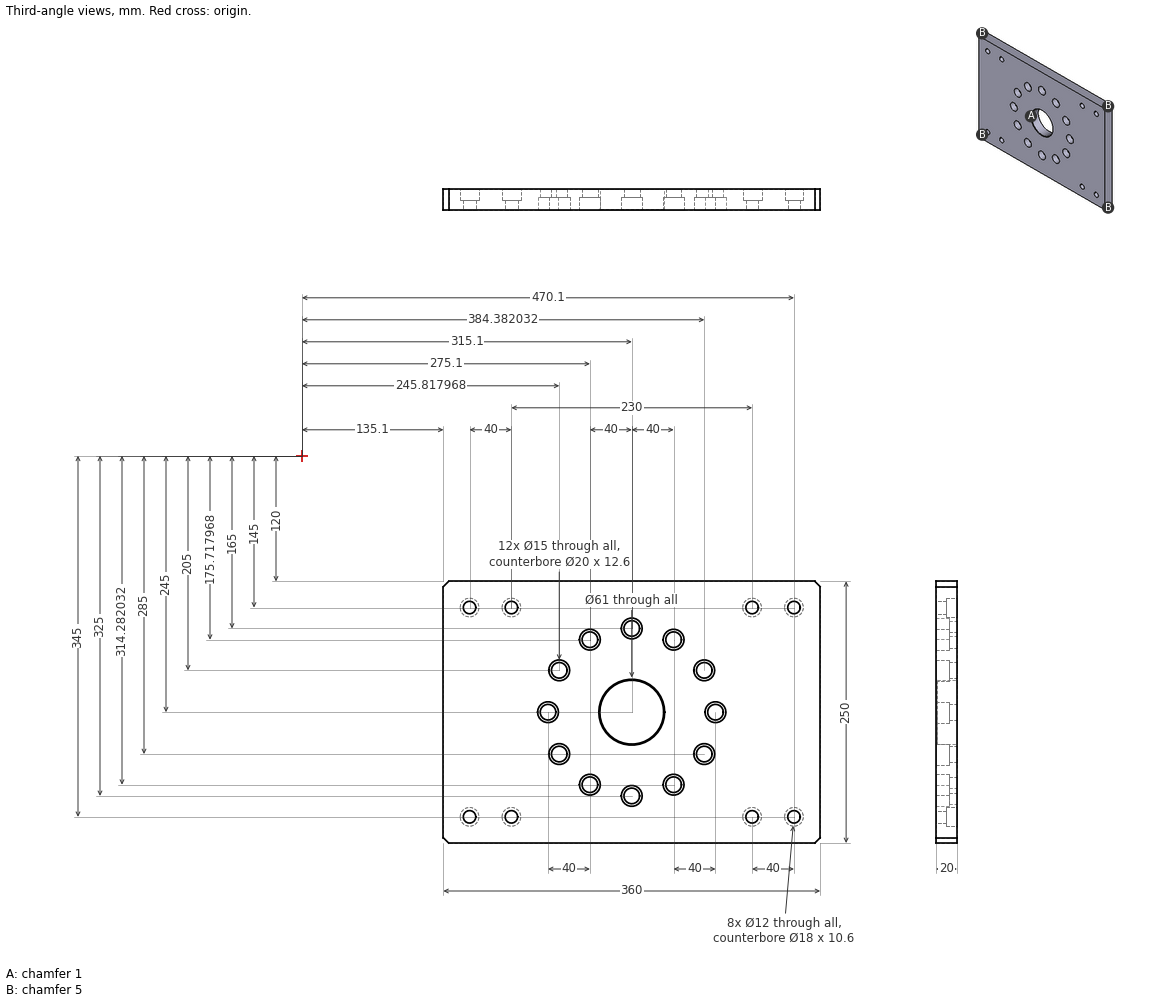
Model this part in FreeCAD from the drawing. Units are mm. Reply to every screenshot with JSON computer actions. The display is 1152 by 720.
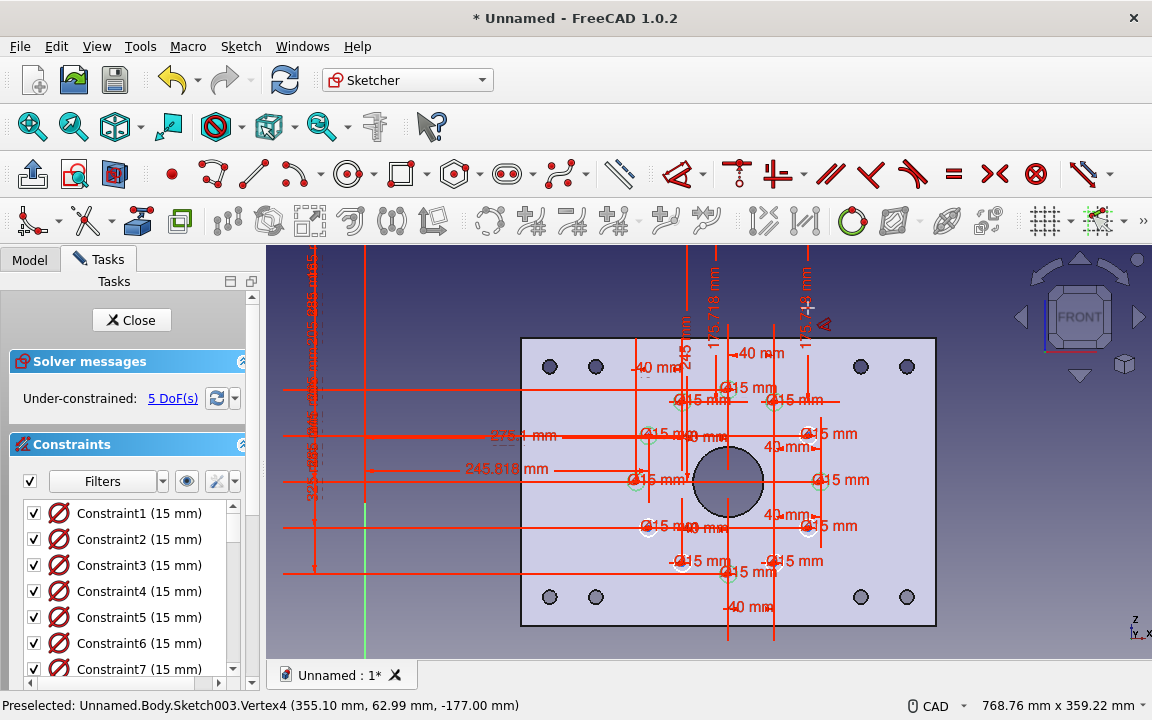
{"action": "left_click", "coordinate": [809, 436]}
{"action": "left_click", "coordinate": [587, 470]}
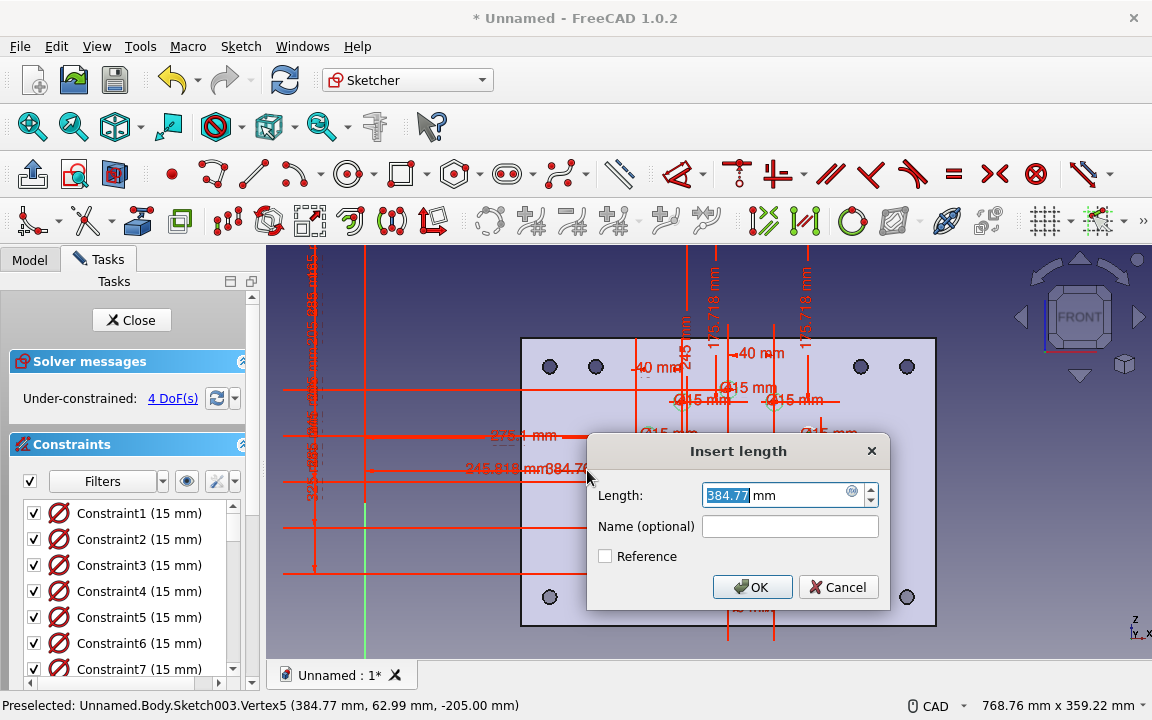
{"action": "type", "text": "384.382032"}
{"action": "key", "text": "Return"}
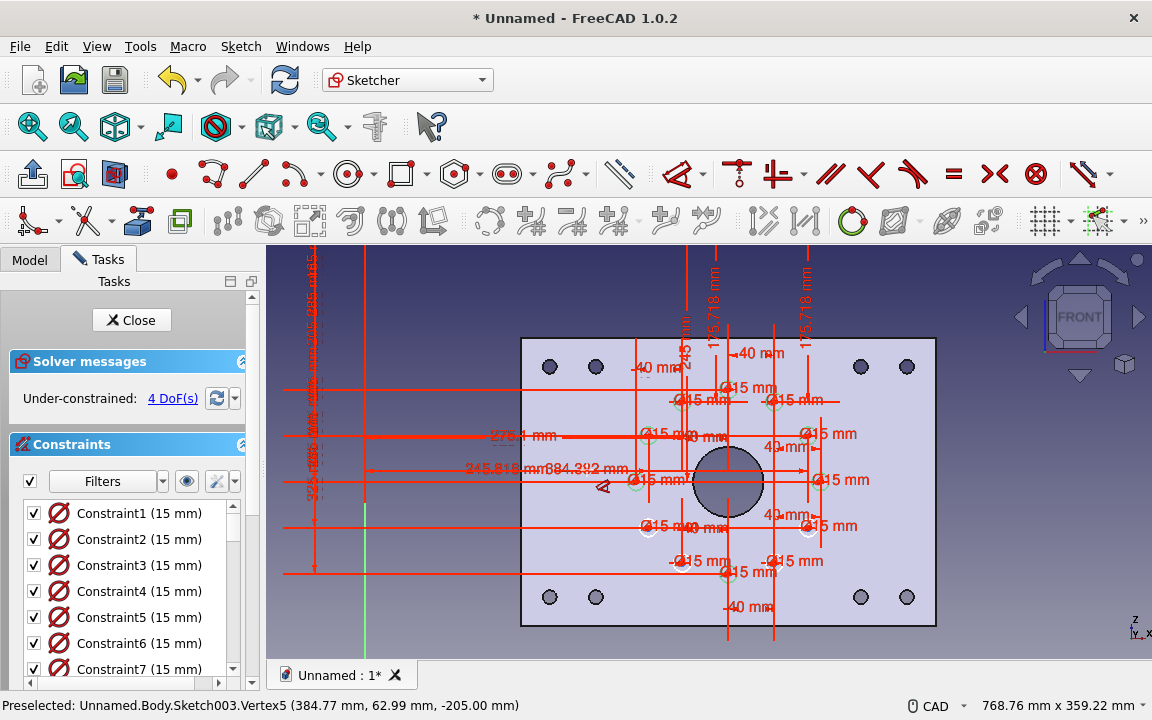
{"action": "left_click", "coordinate": [809, 528]}
{"action": "left_click", "coordinate": [587, 562]}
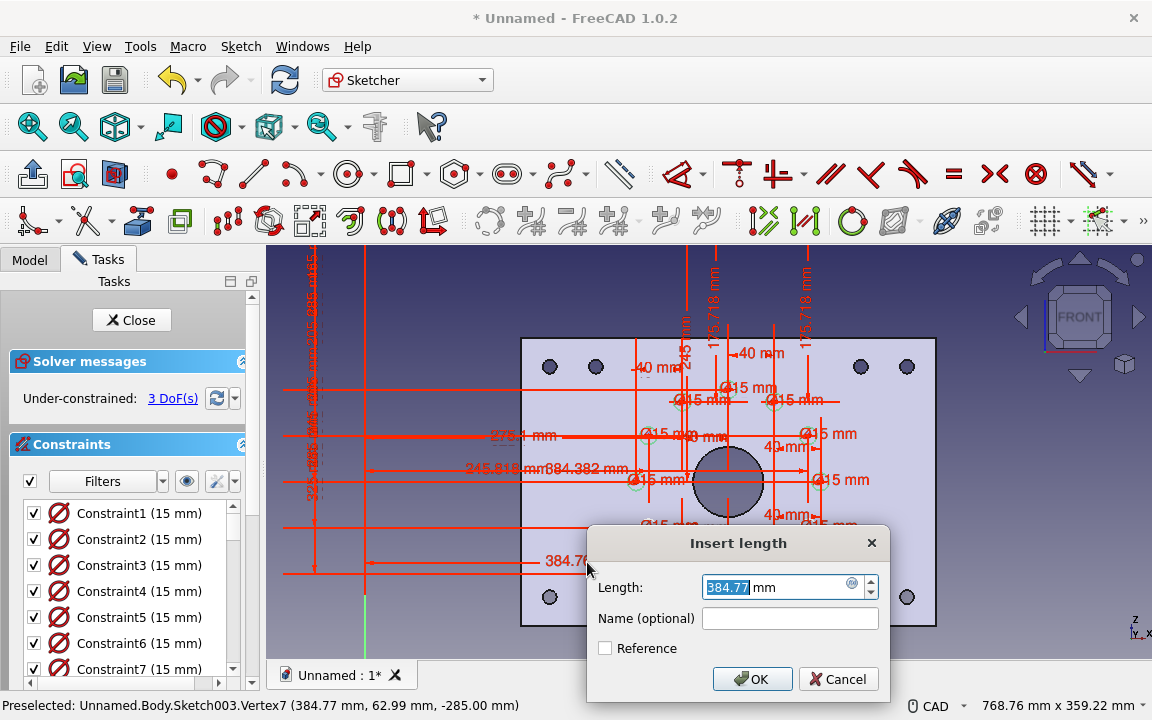
{"action": "type", "text": "384.382032"}
{"action": "key", "text": "Return"}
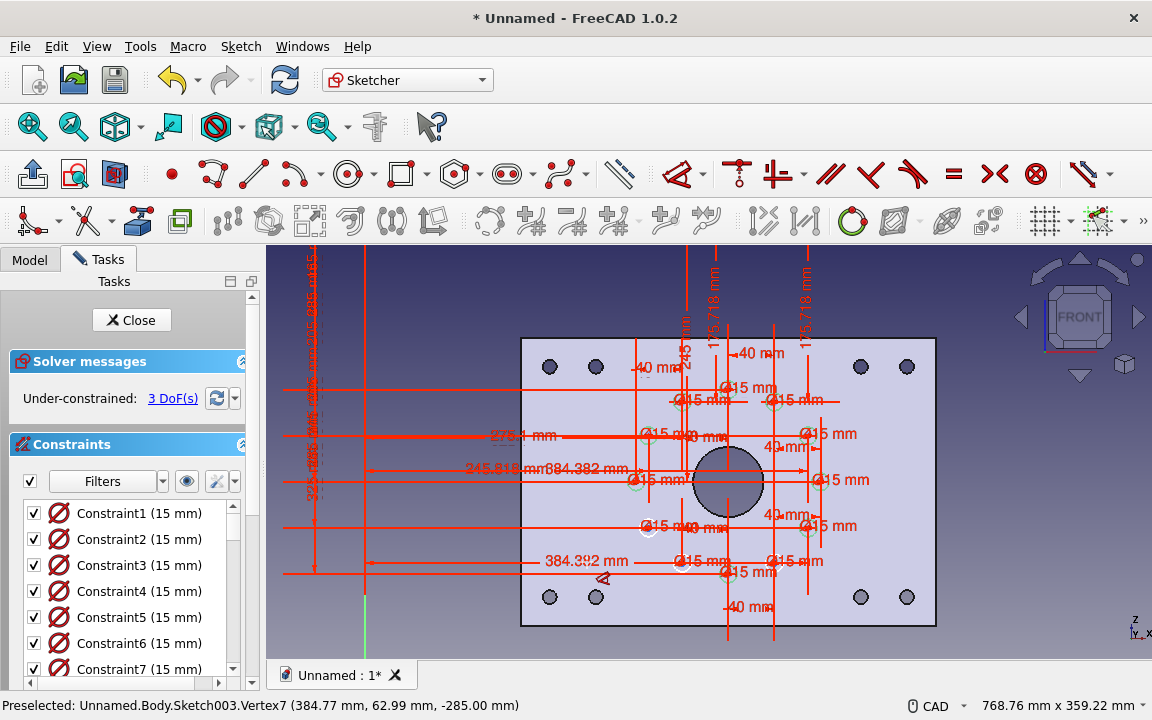
{"action": "left_click", "coordinate": [774, 563]}
{"action": "left_click", "coordinate": [331, 351]}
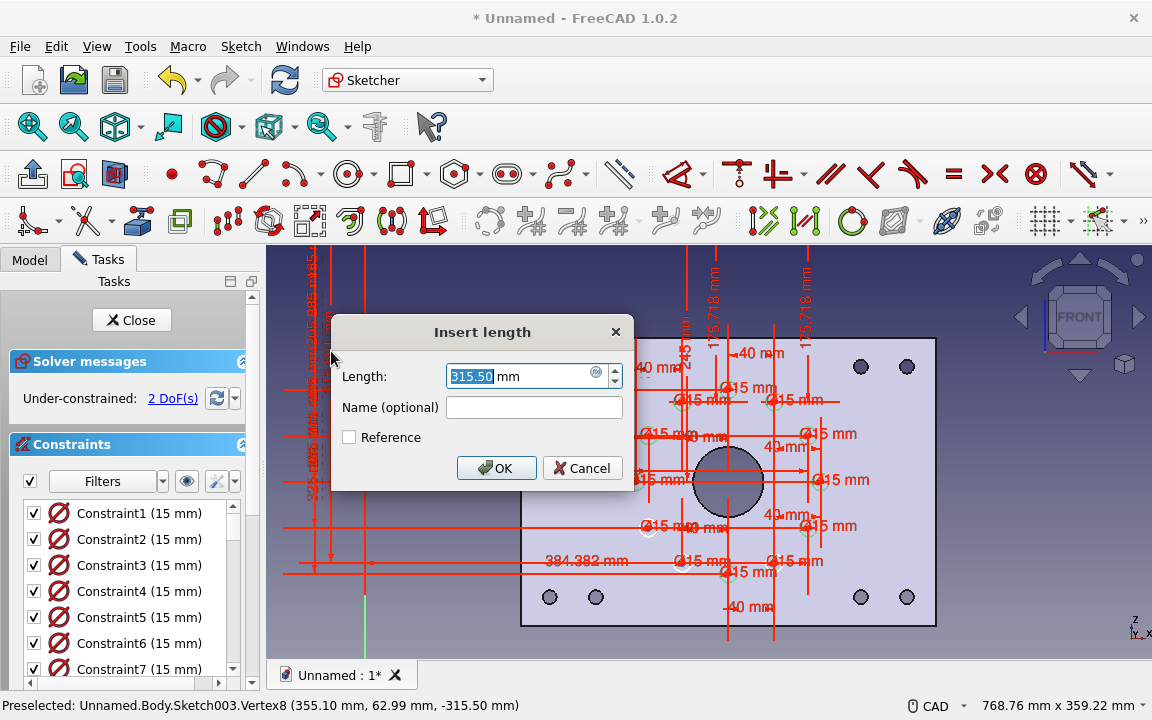
{"action": "type", "text": "314.282032"}
{"action": "key", "text": "Return"}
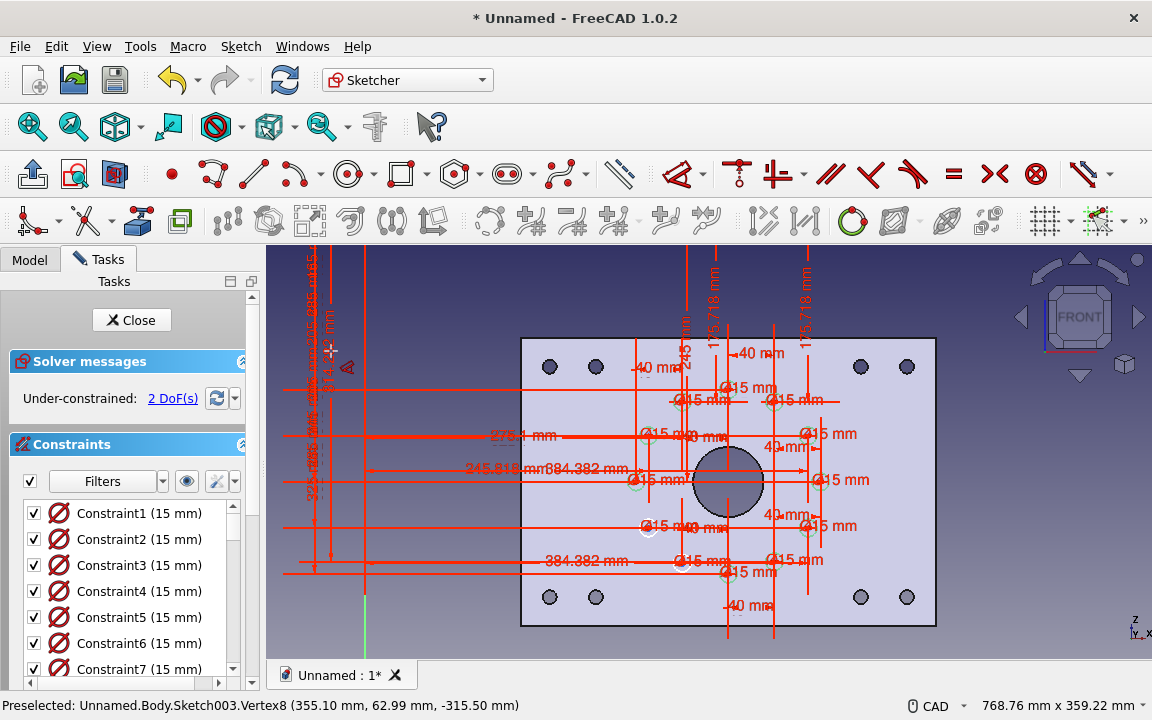
{"action": "left_click", "coordinate": [682, 563]}
{"action": "left_click", "coordinate": [331, 520]}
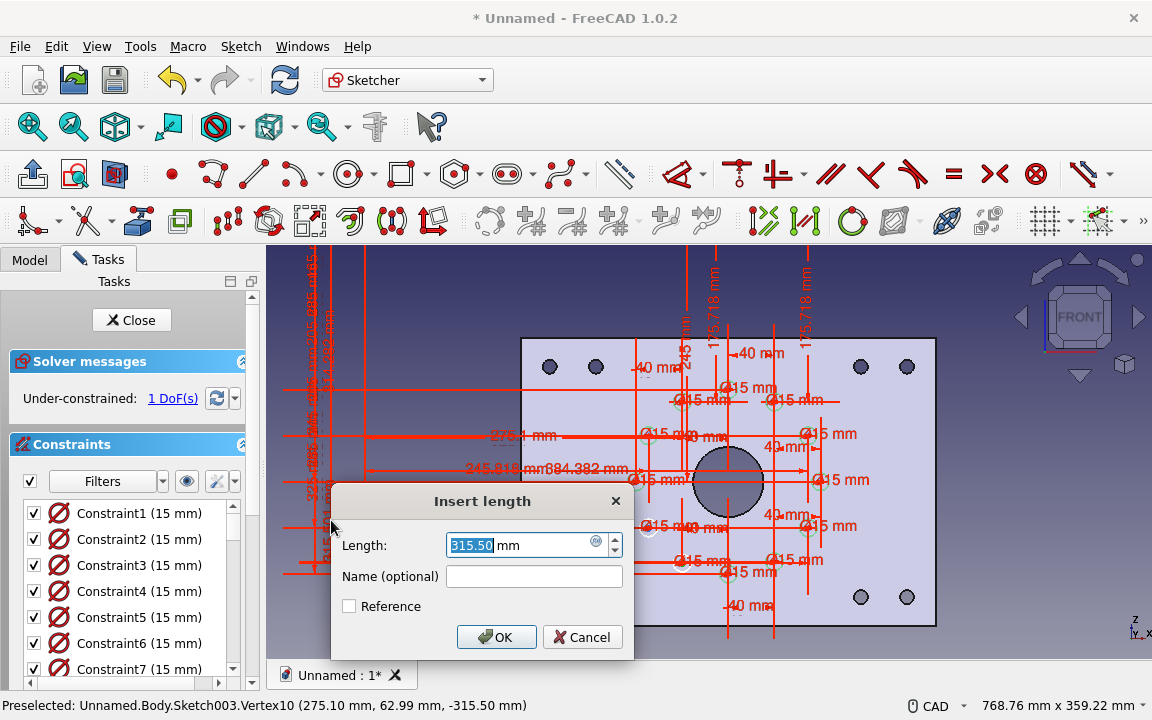
{"action": "type", "text": "314.282032"}
{"action": "key", "text": "Return"}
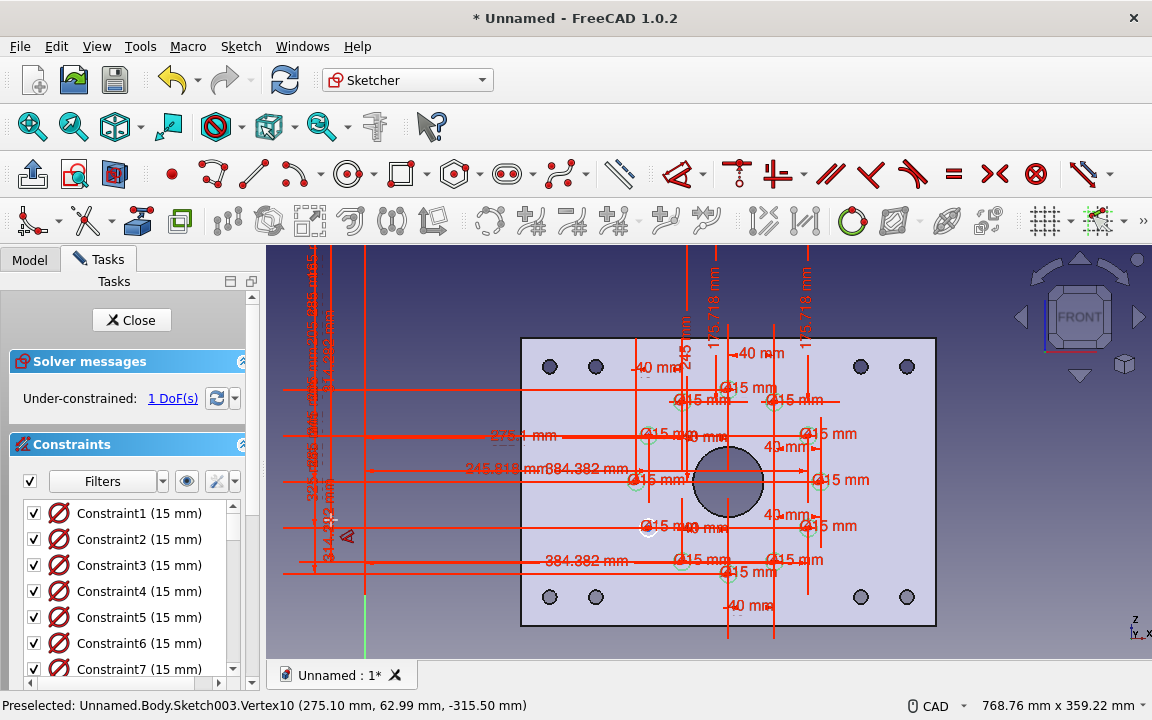
{"action": "left_click", "coordinate": [649, 528]}
{"action": "left_click", "coordinate": [507, 562]}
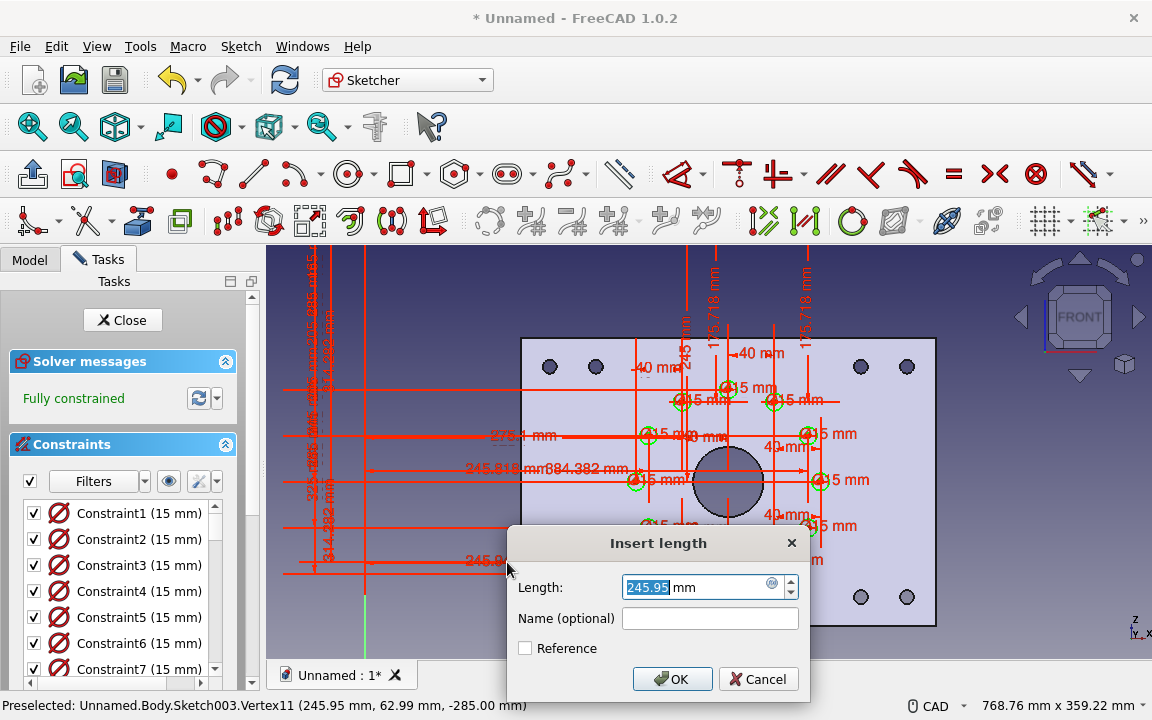
{"action": "type", "text": "245.817968"}
{"action": "key", "text": "Return"}
{"action": "key", "text": "Escape"}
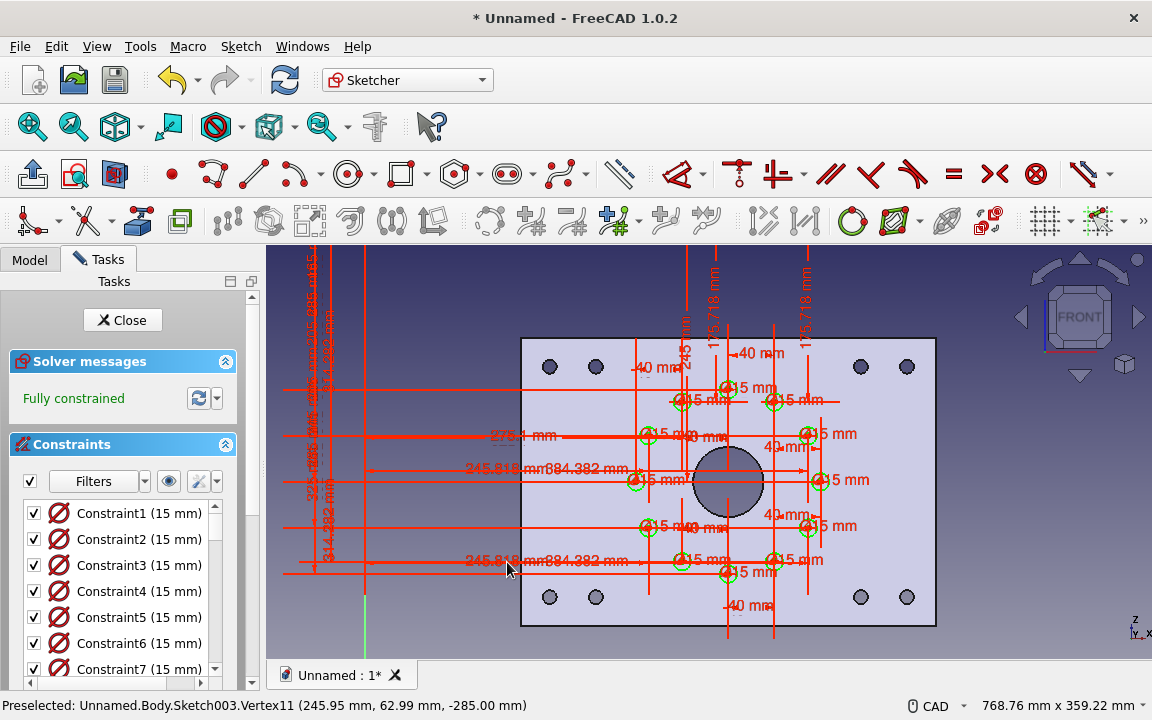
{"action": "left_click", "coordinate": [123, 320]}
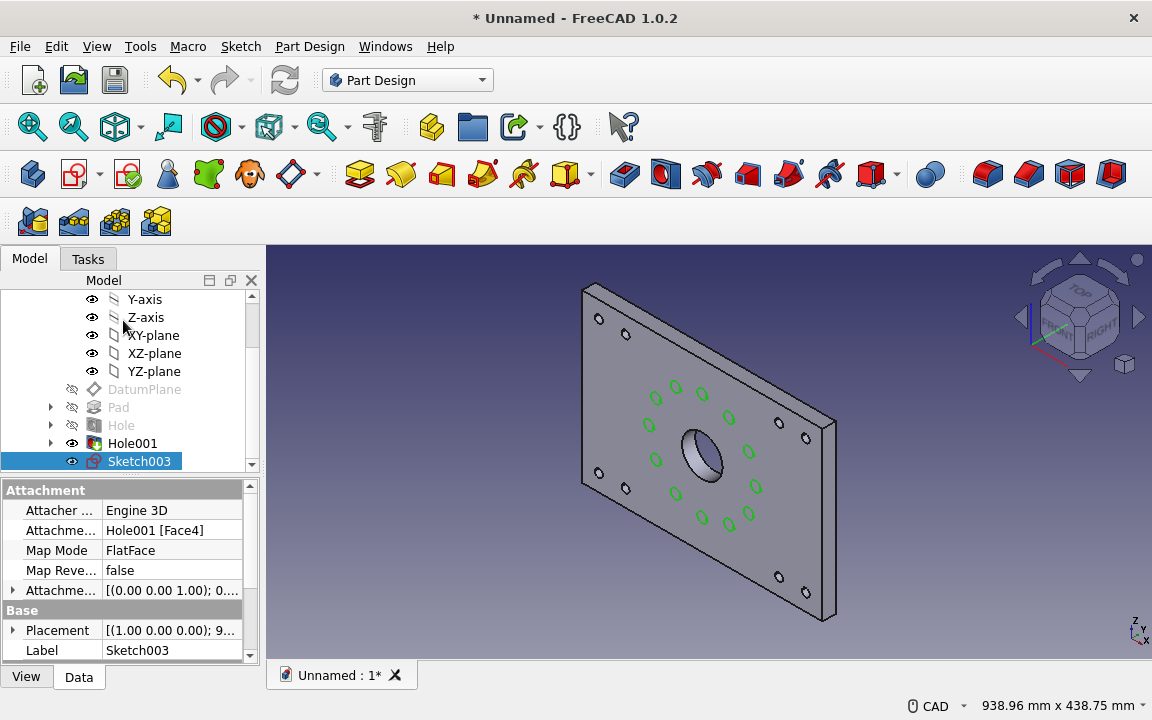
{"action": "left_click", "coordinate": [666, 174]}